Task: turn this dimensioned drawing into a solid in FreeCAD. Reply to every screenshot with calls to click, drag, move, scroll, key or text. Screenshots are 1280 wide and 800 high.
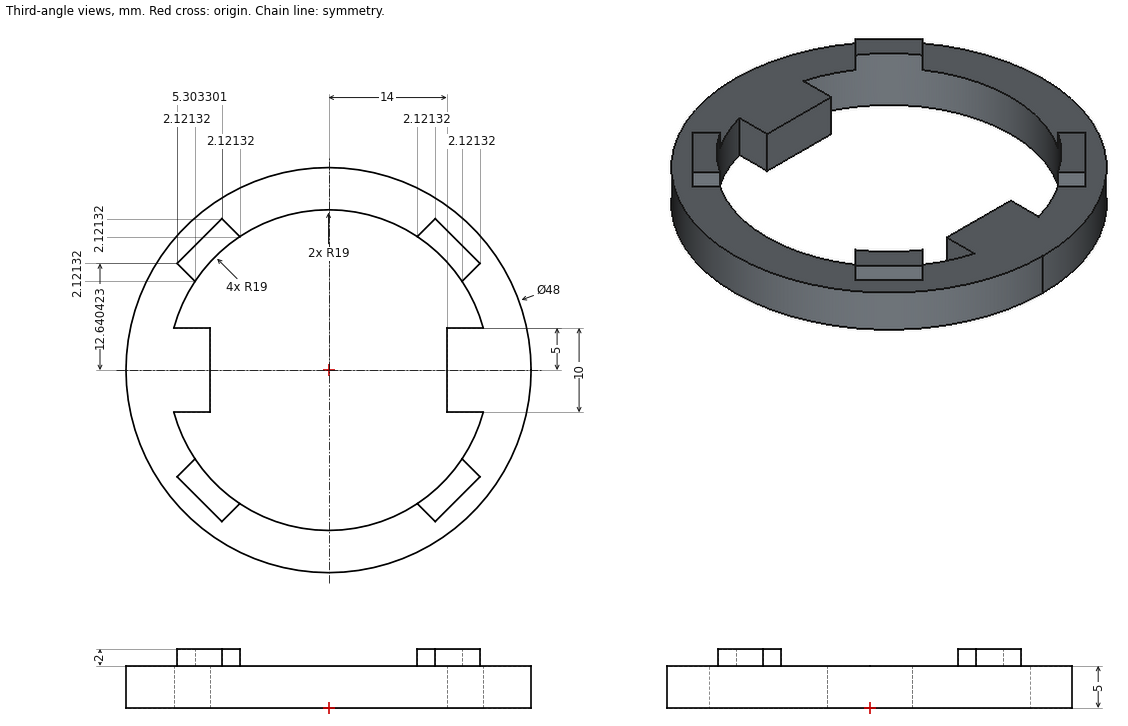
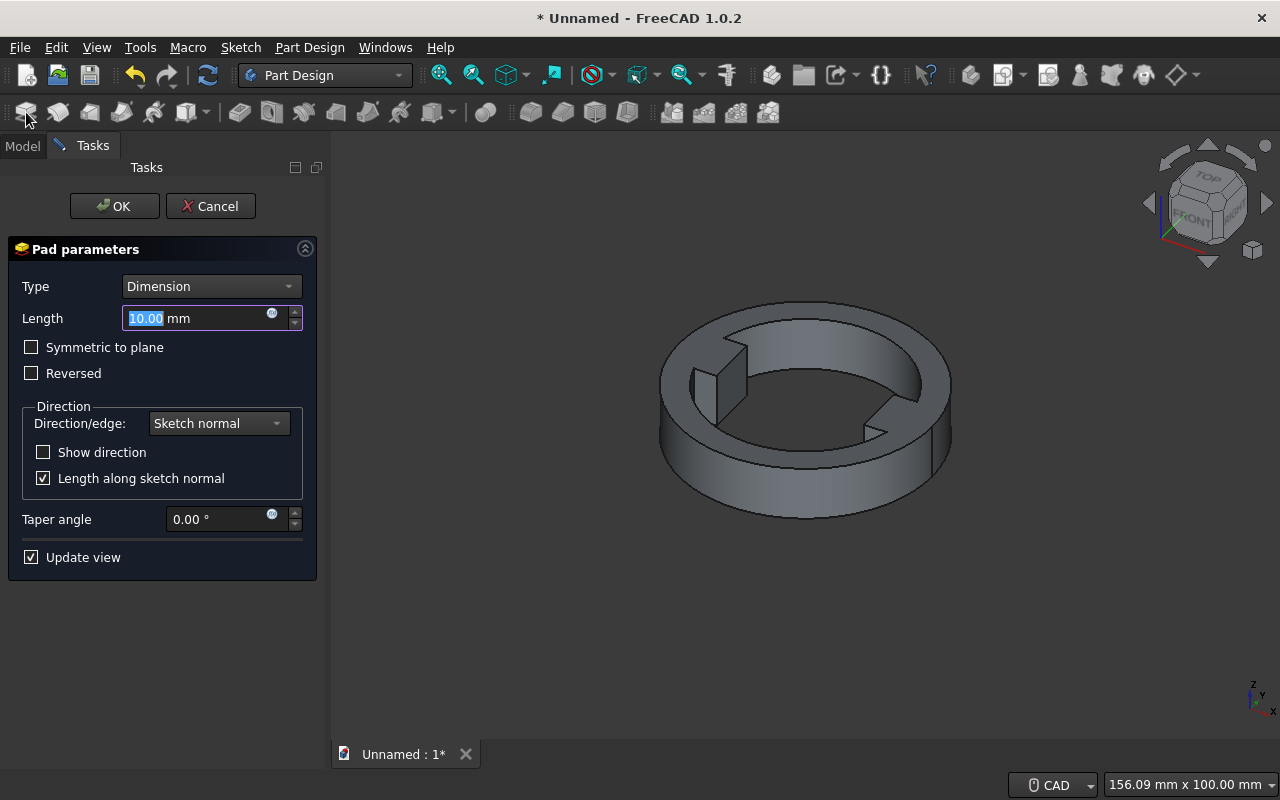
text(5)
key(Tab)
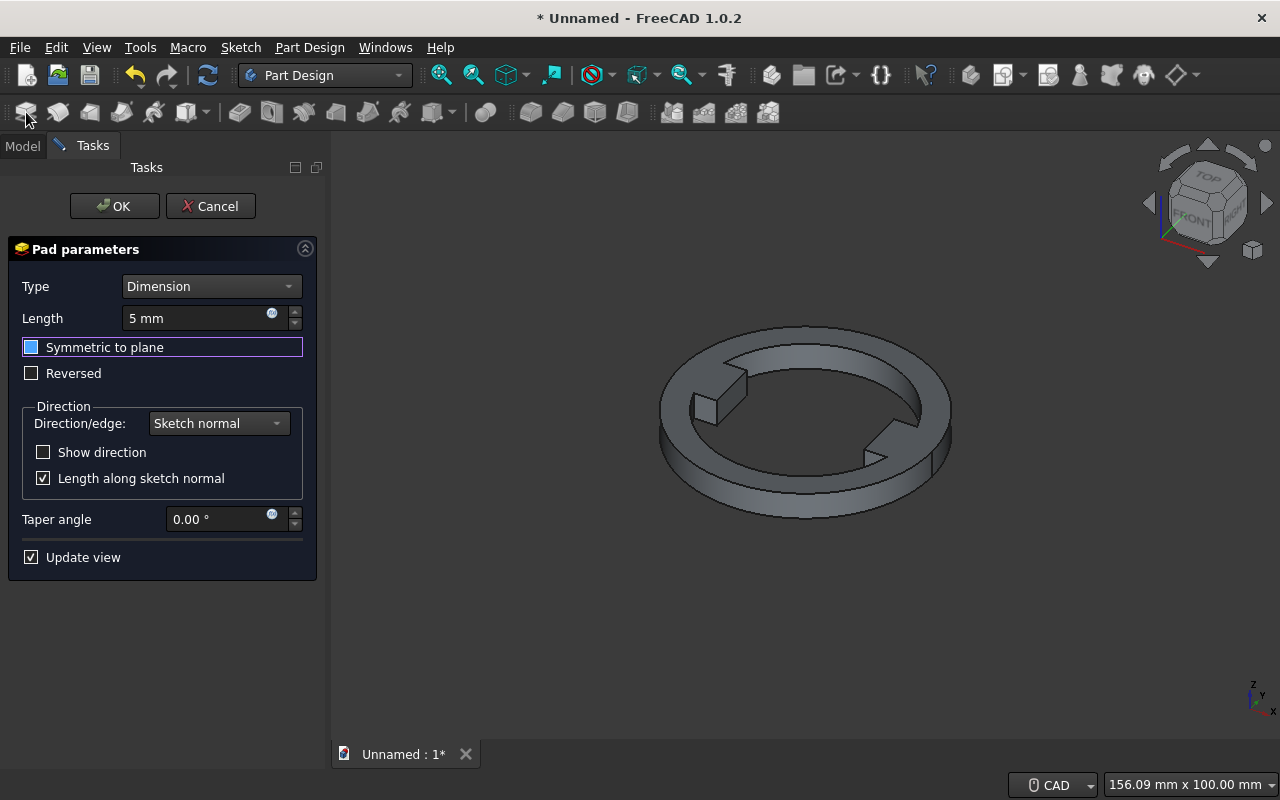
click(115, 206)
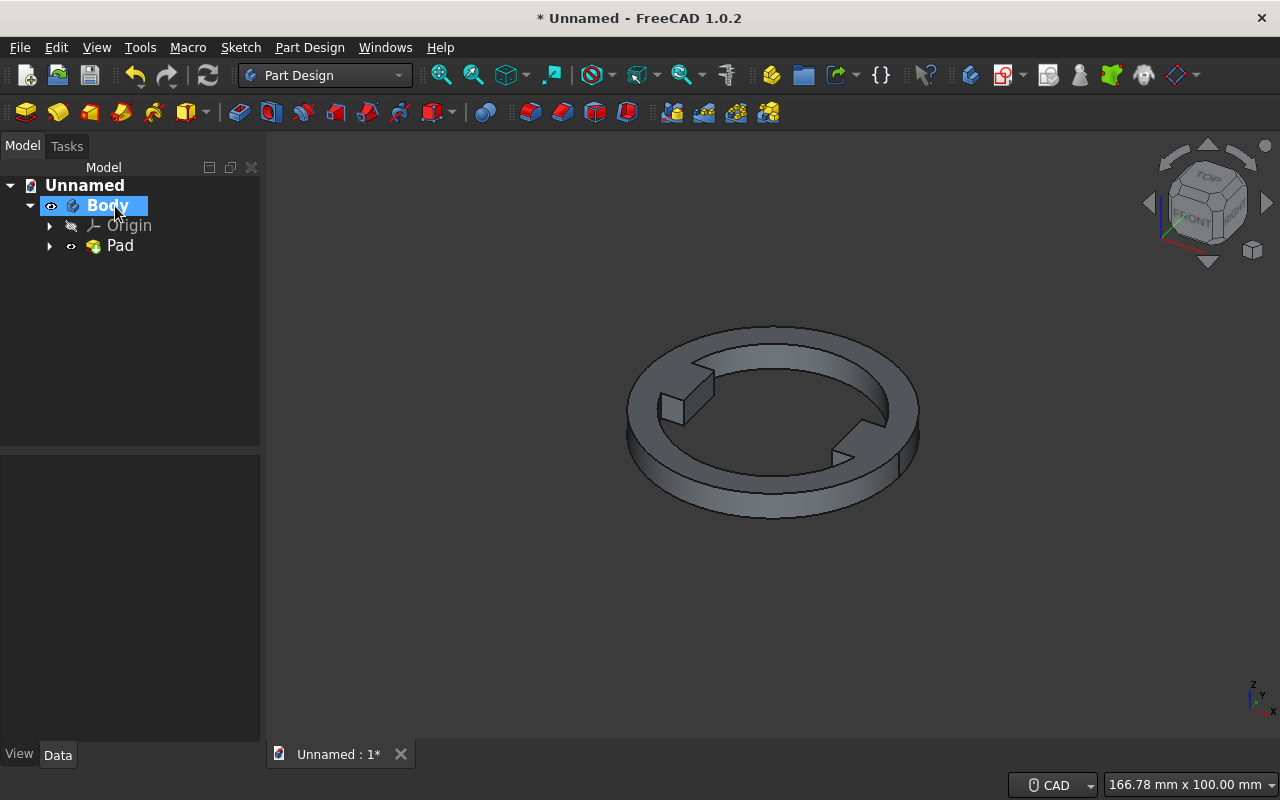
key(v)
key(f)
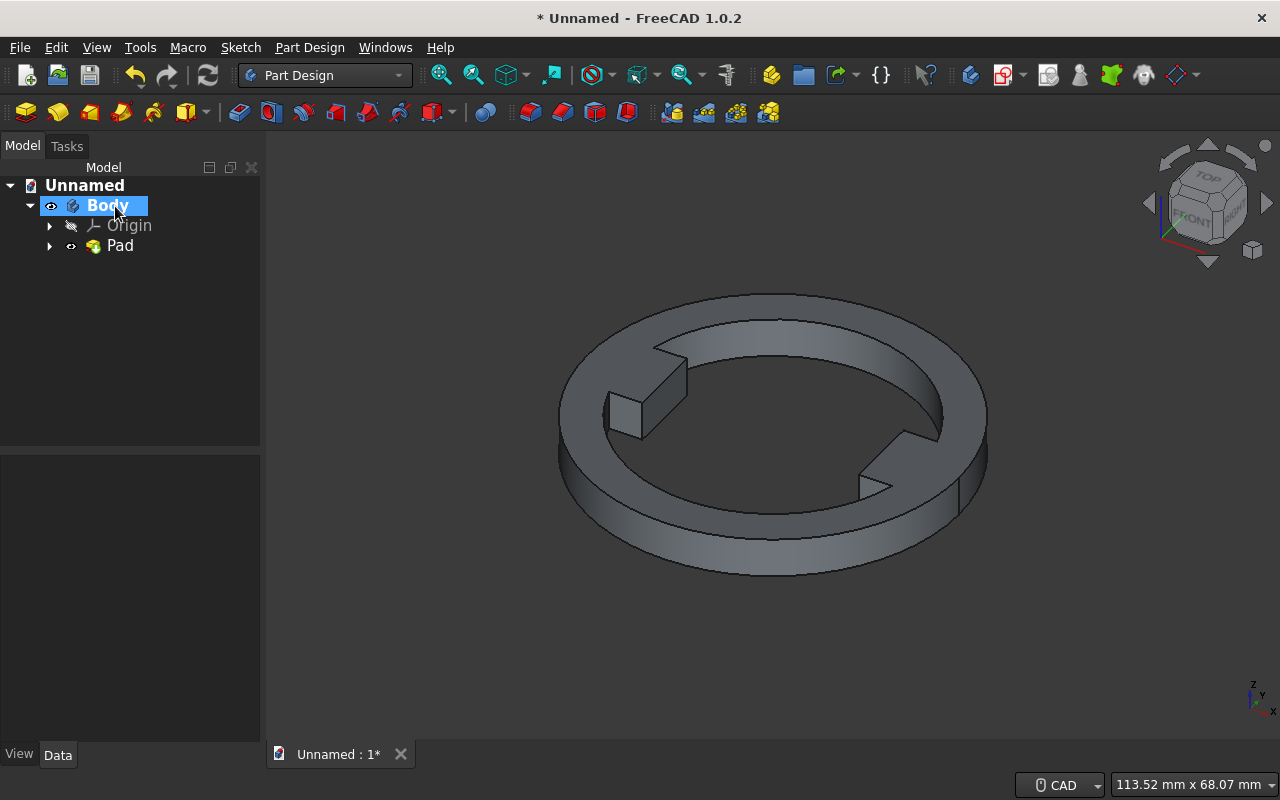
click(932, 468)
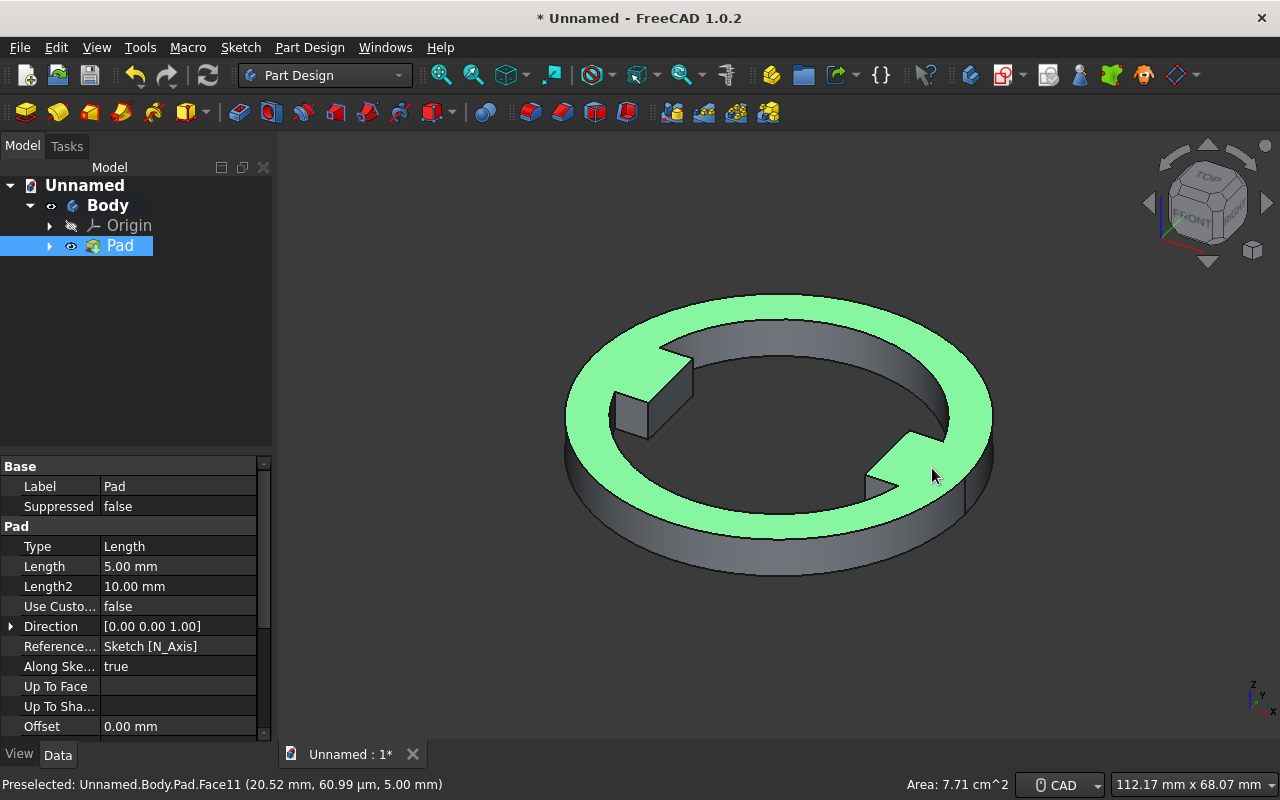
click(1004, 76)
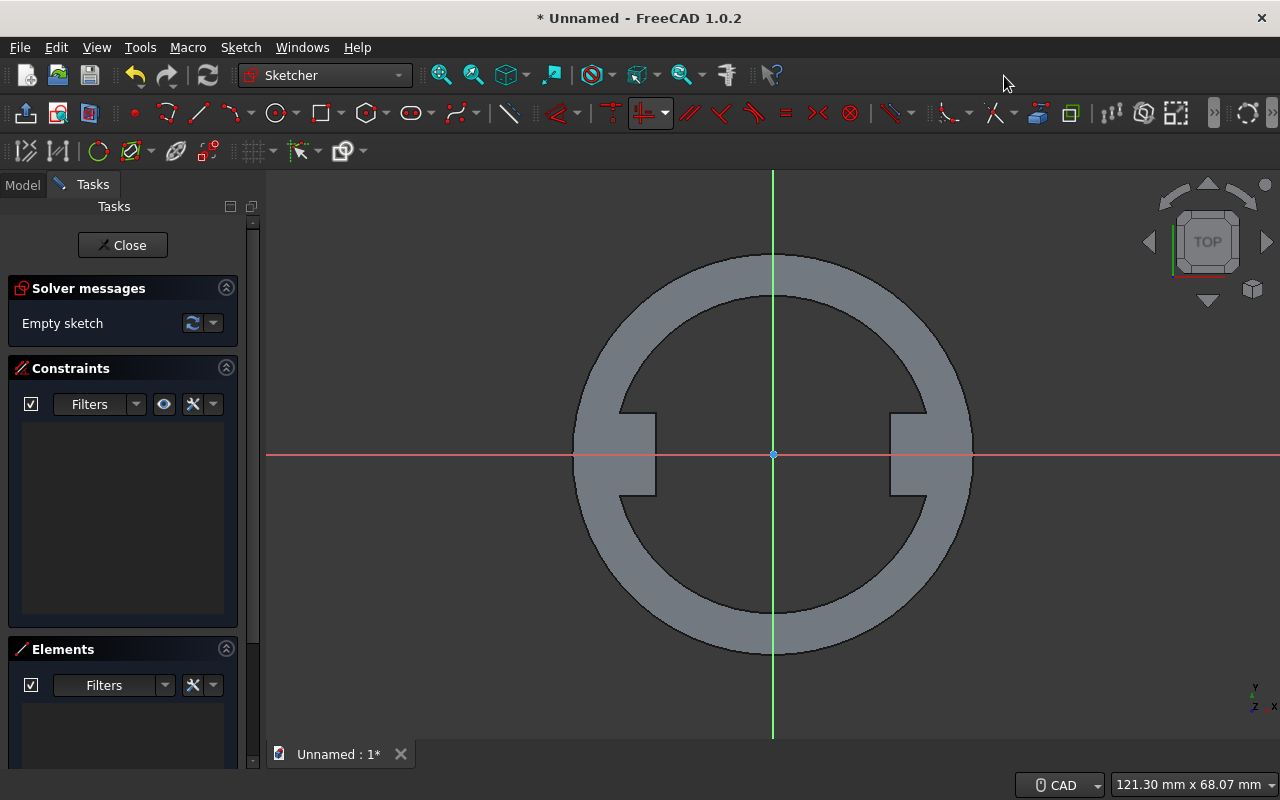
click(168, 114)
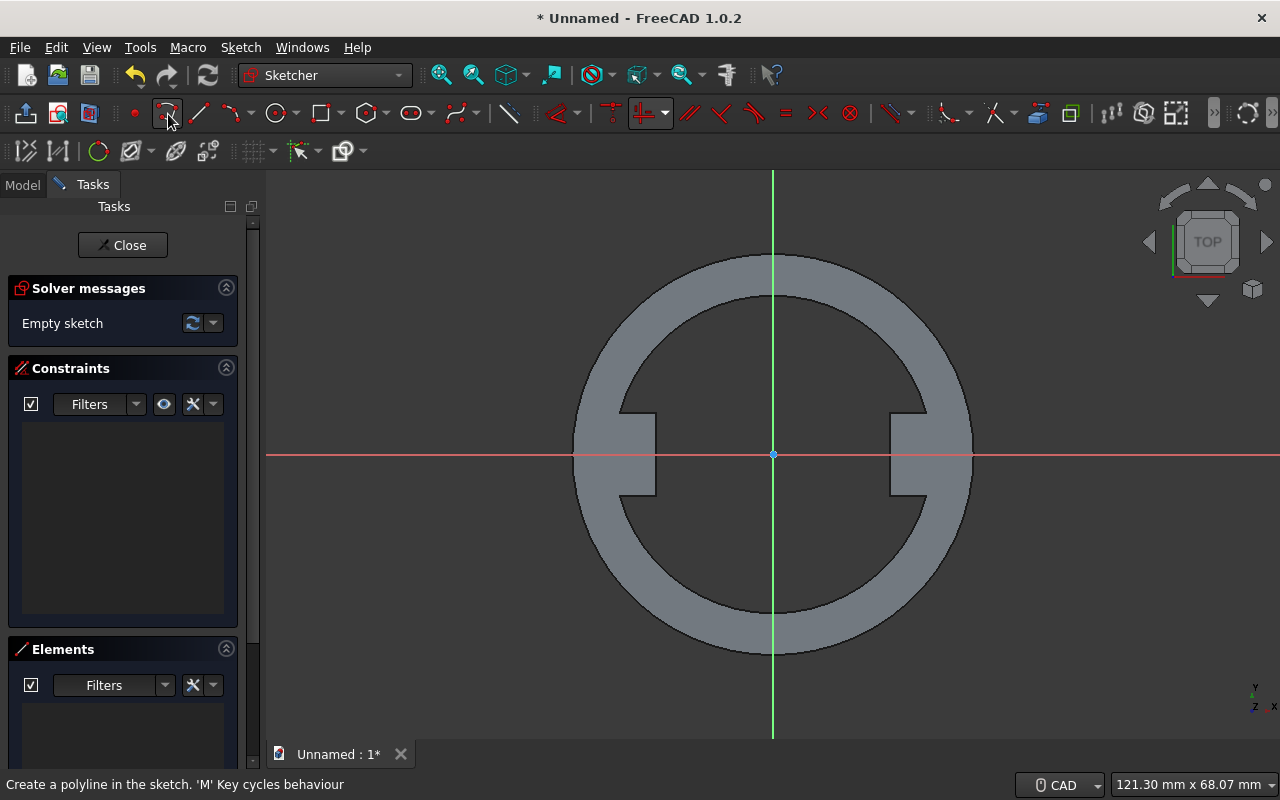
click(685, 322)
click(667, 304)
click(623, 349)
click(641, 367)
right_click(641, 367)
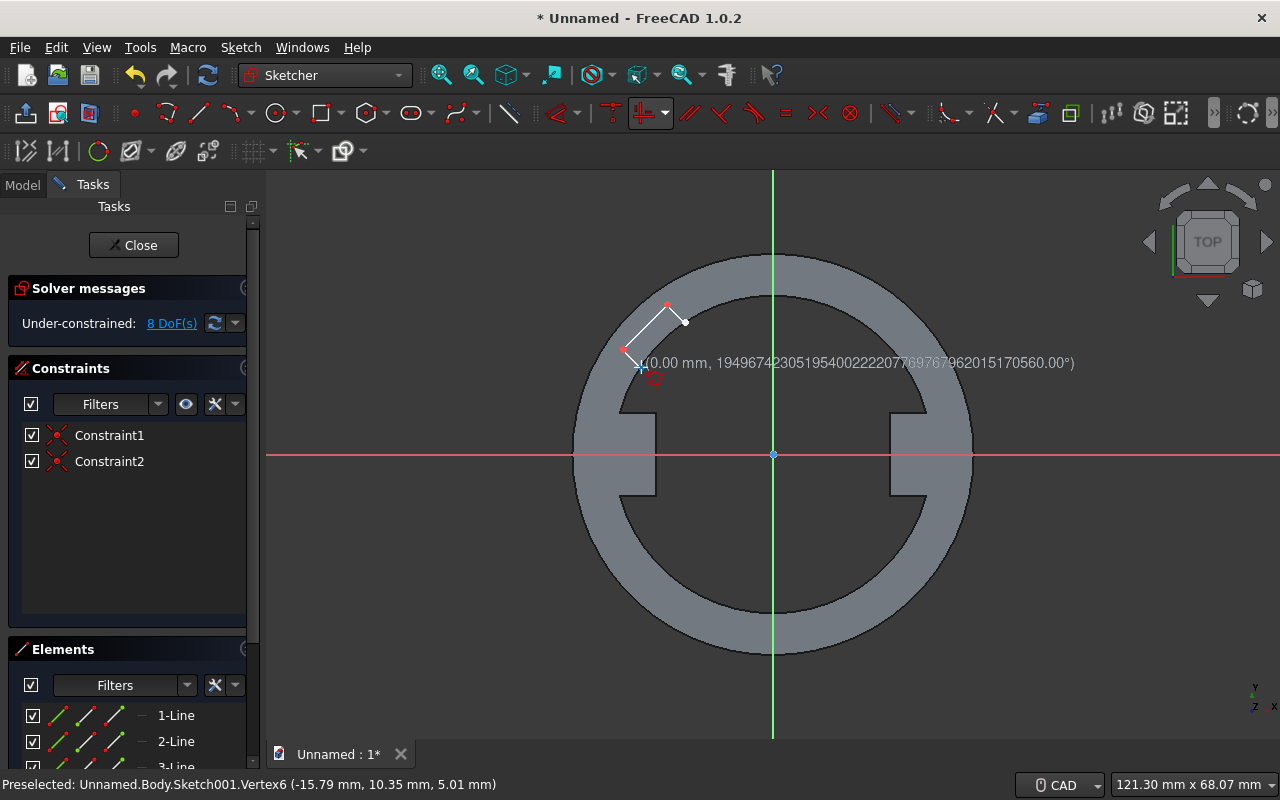
key(g)
key(3)
key(a)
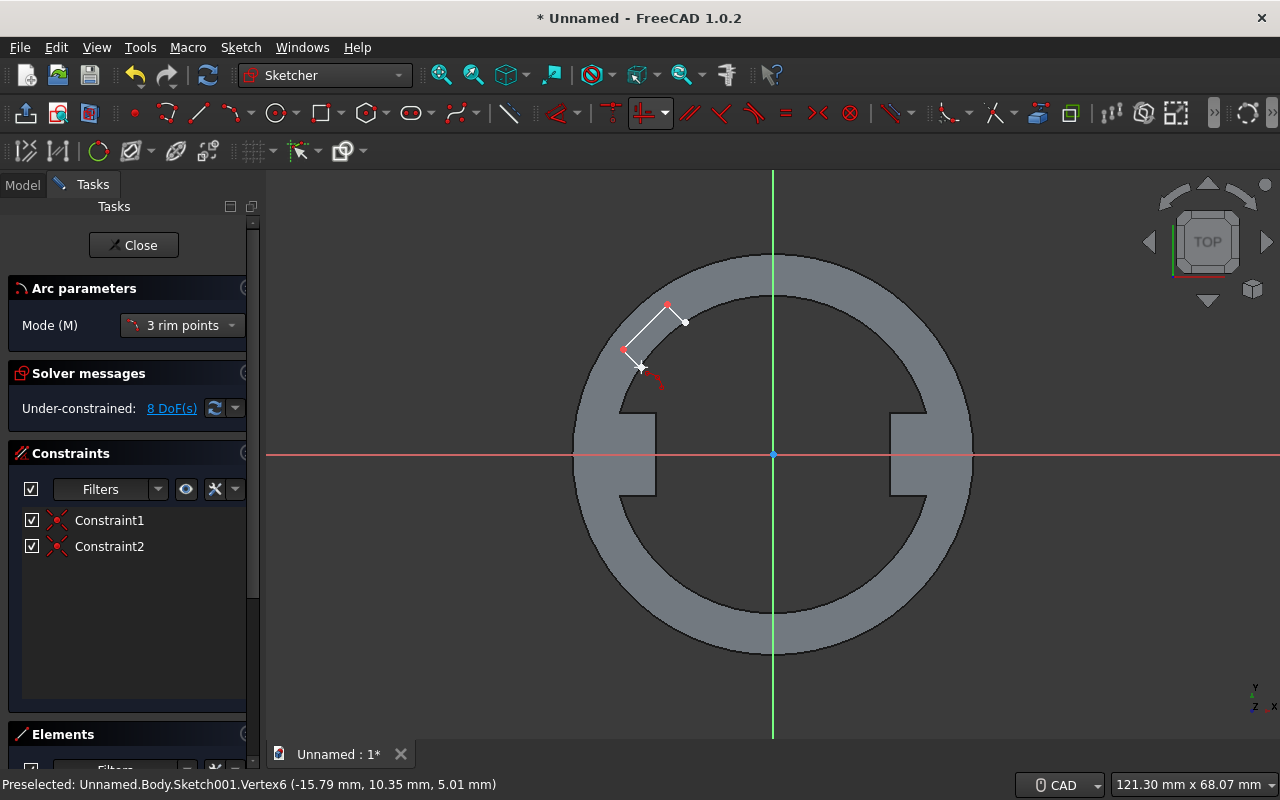
scroll(641, 367, up, 2)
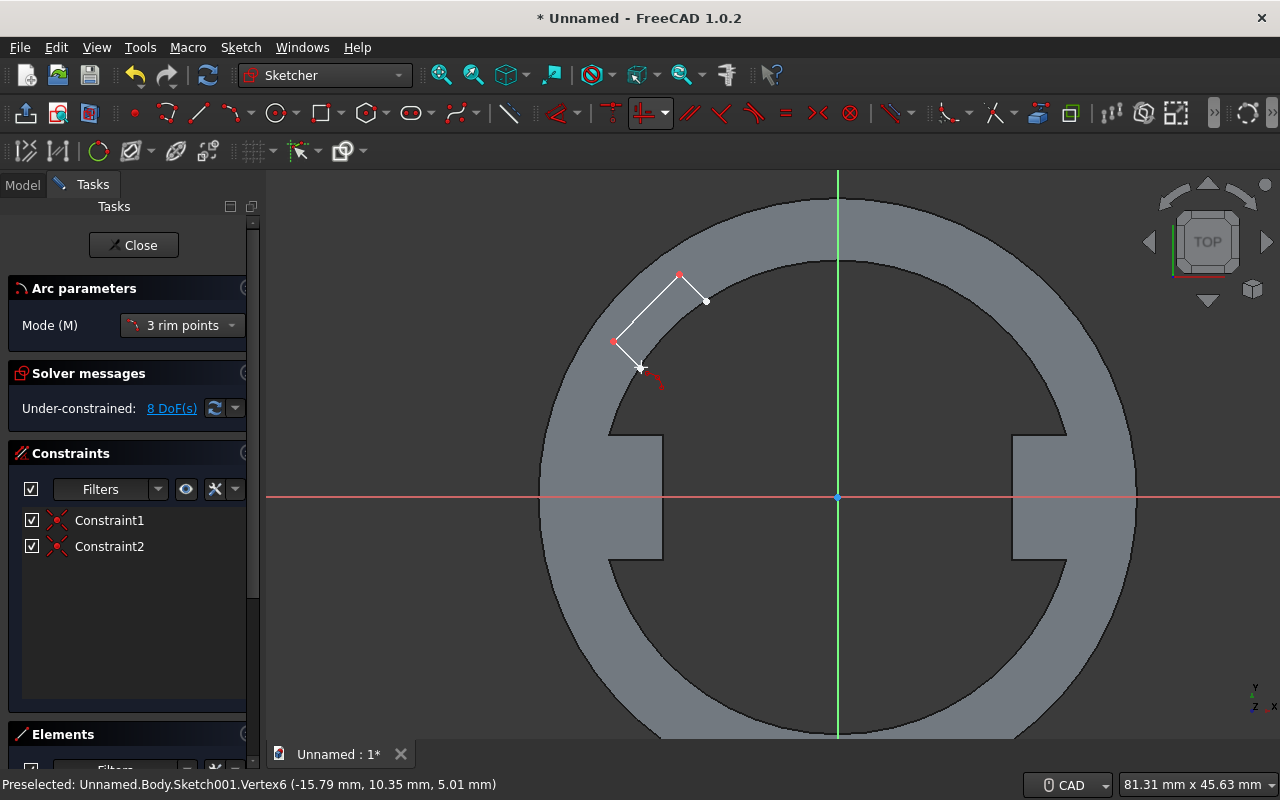
click(641, 368)
click(706, 301)